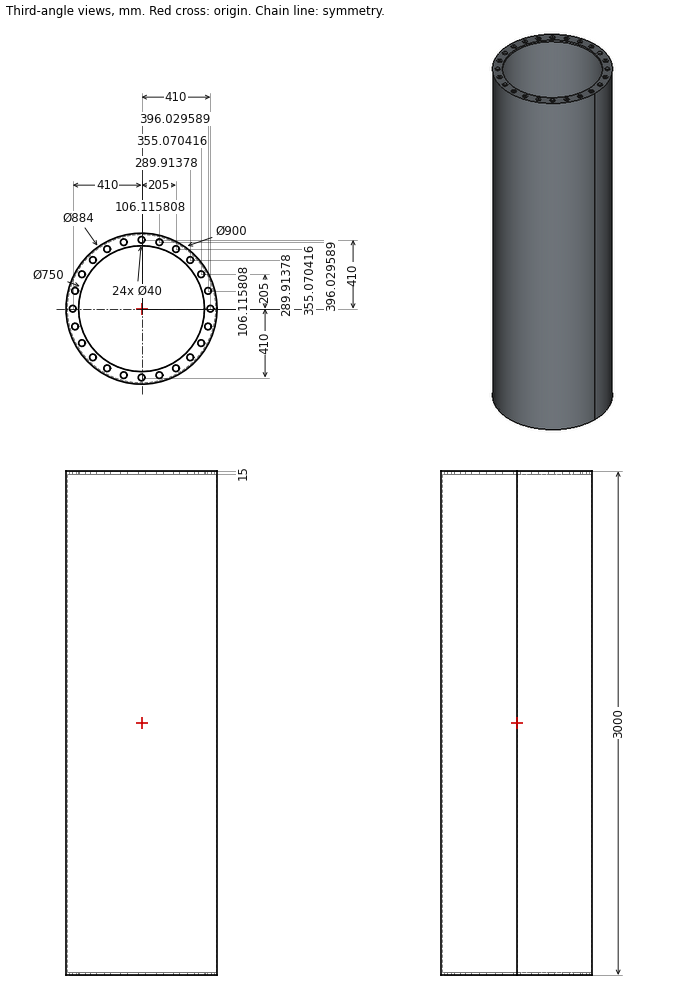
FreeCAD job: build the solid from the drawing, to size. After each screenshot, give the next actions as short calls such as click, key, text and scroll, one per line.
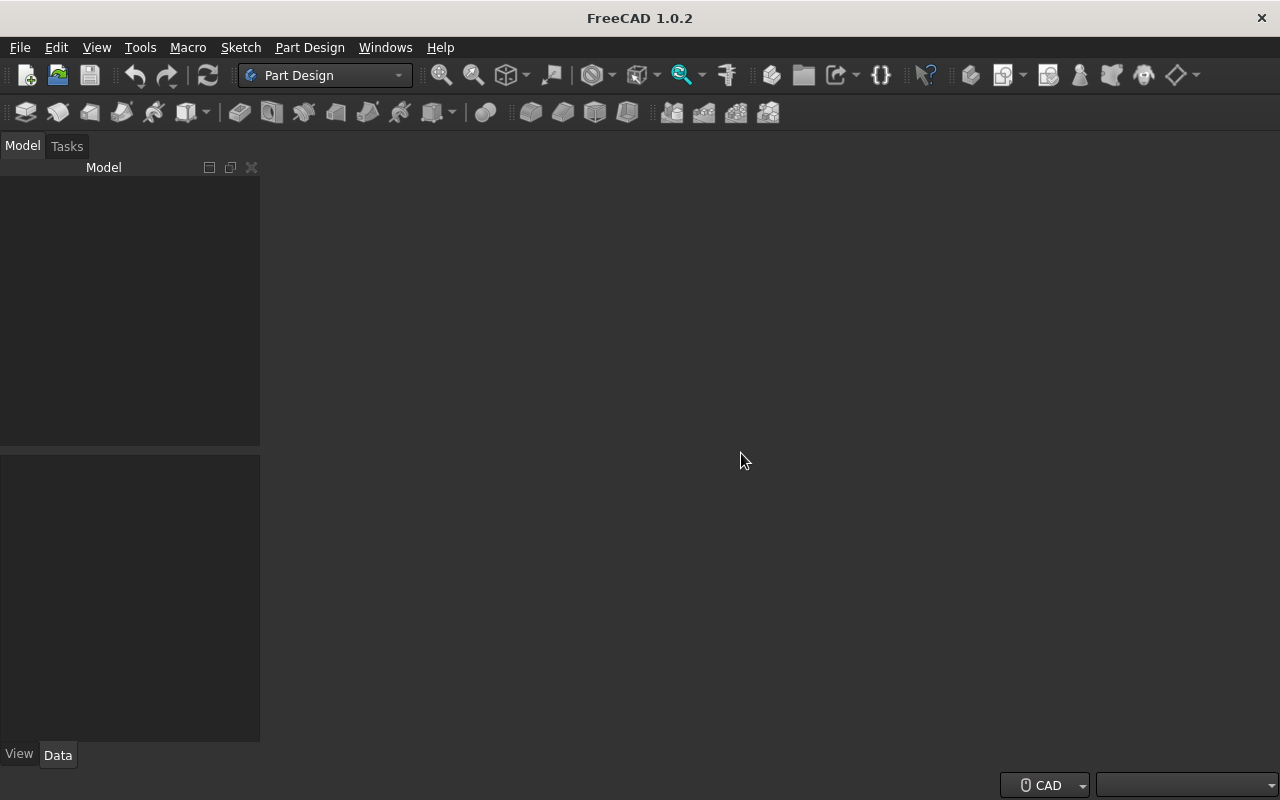
click(26, 76)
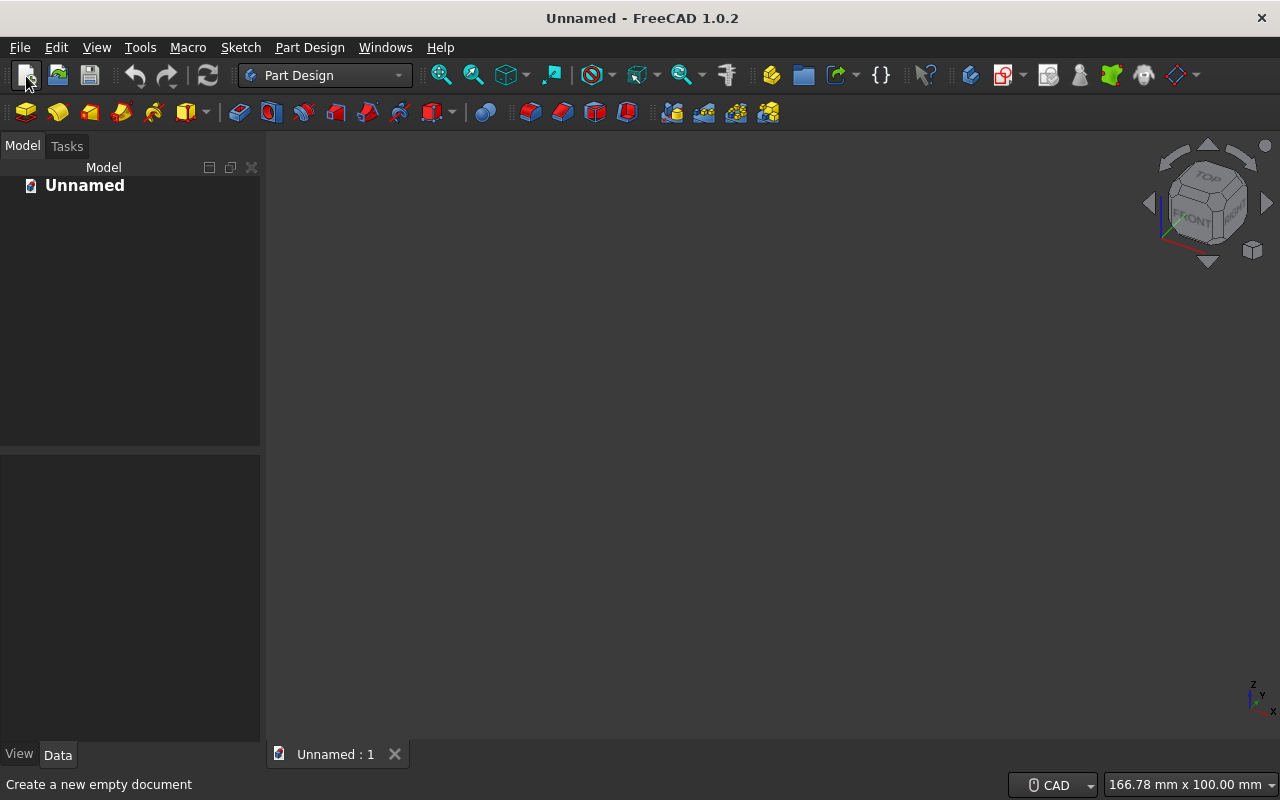
click(1004, 76)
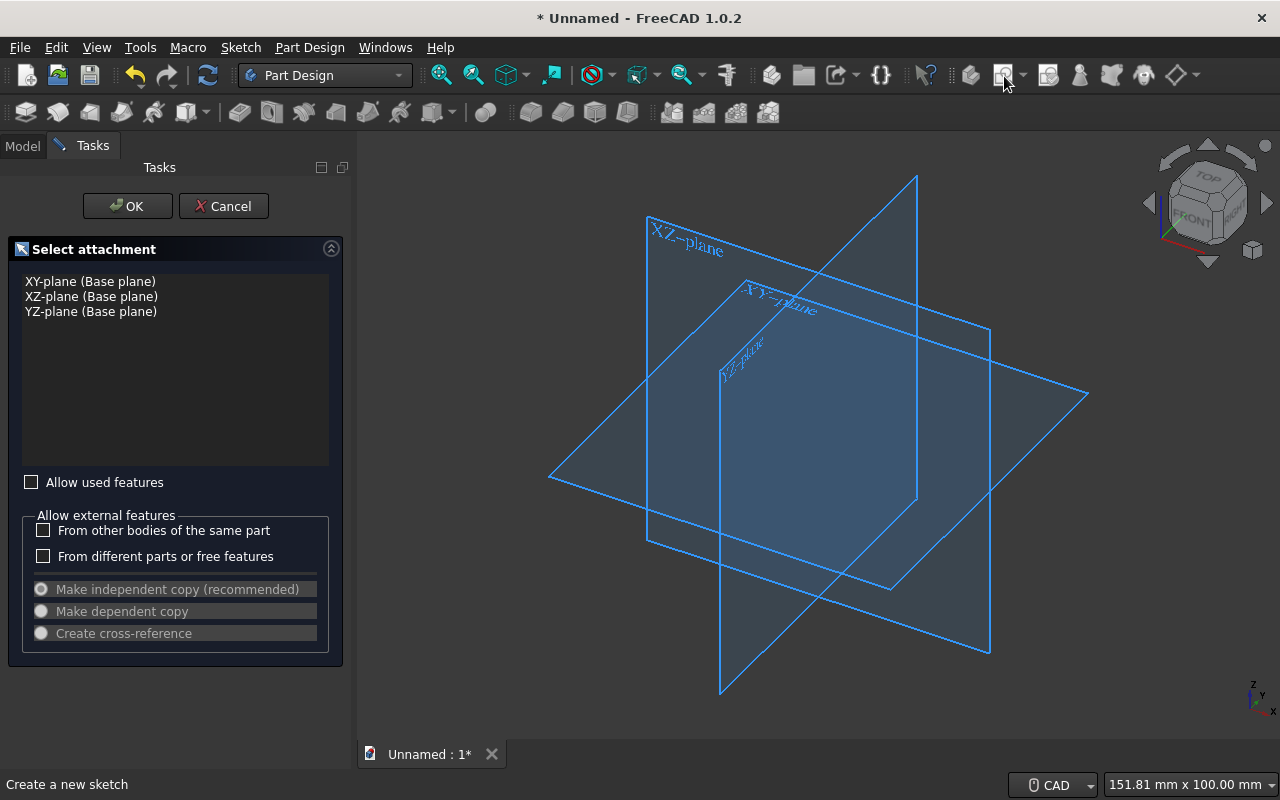
click(82, 282)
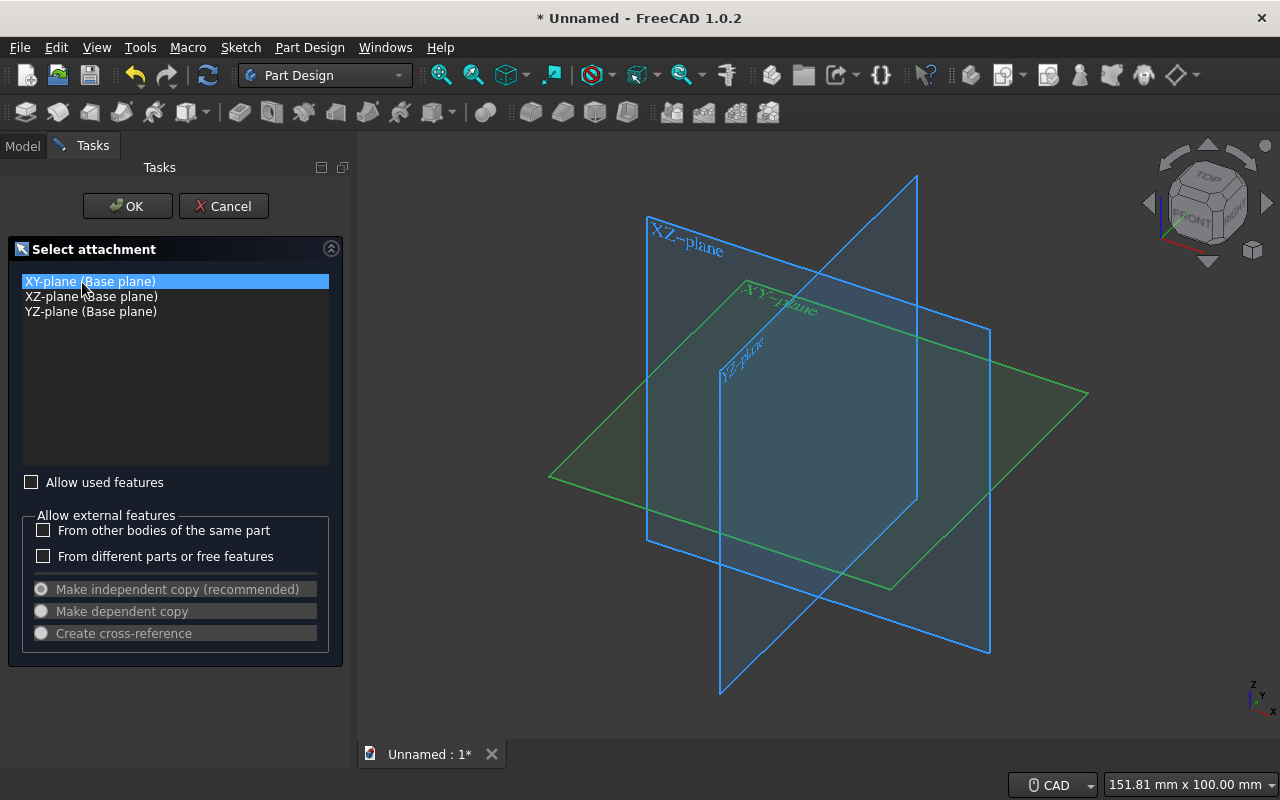
click(128, 206)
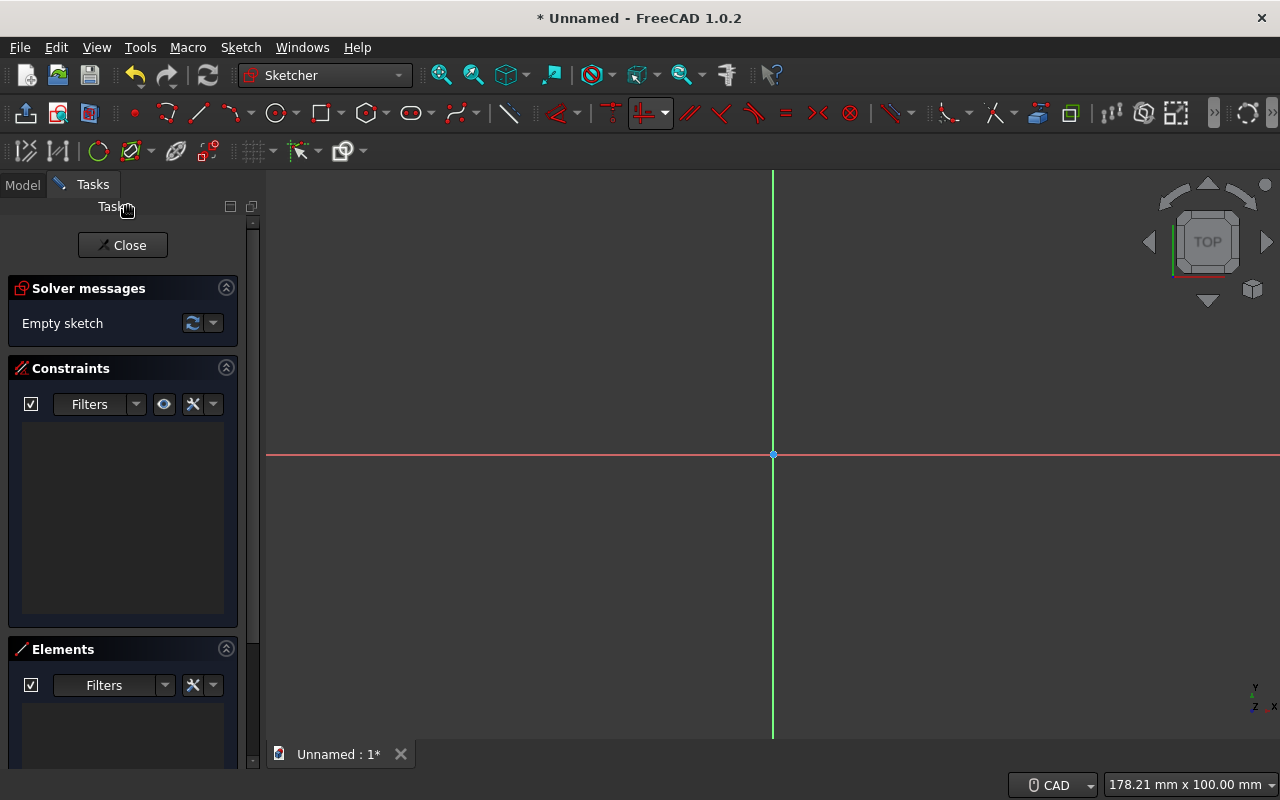
scroll(699, 454, down, 13)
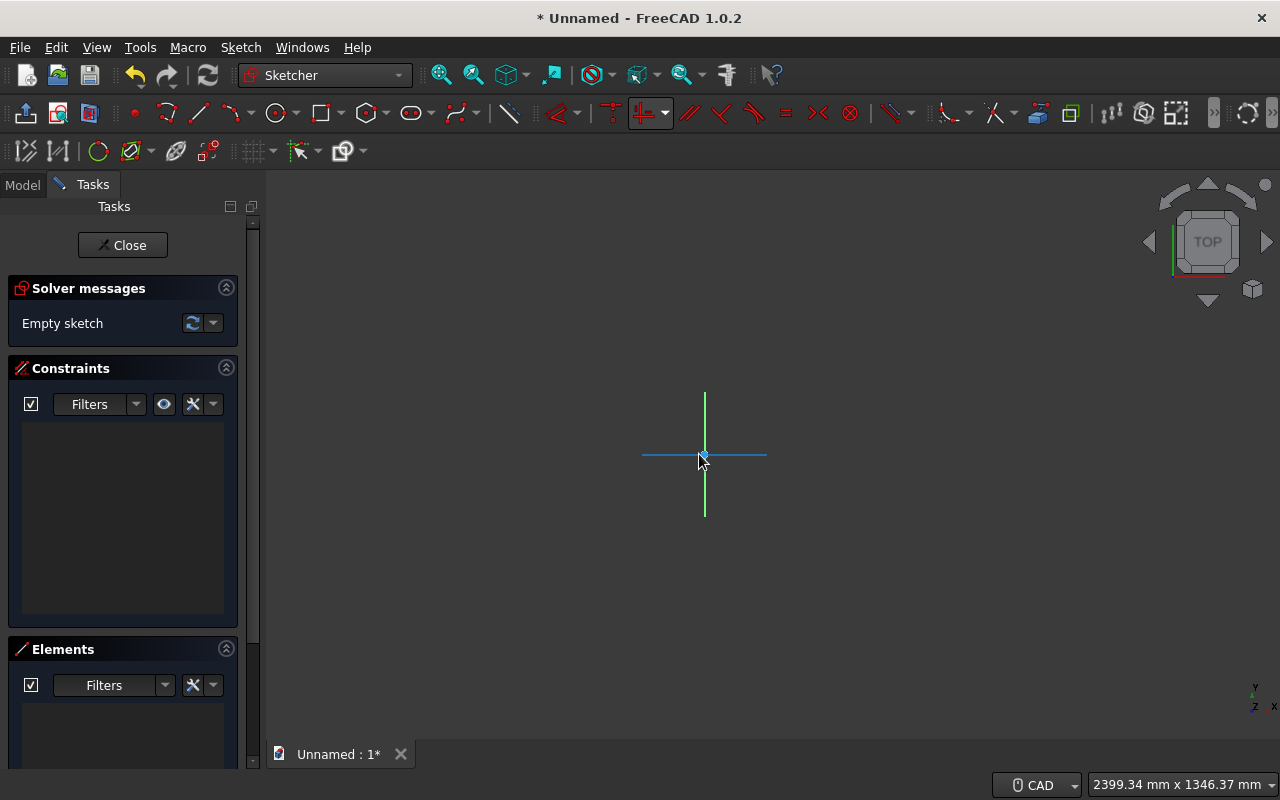
click(276, 114)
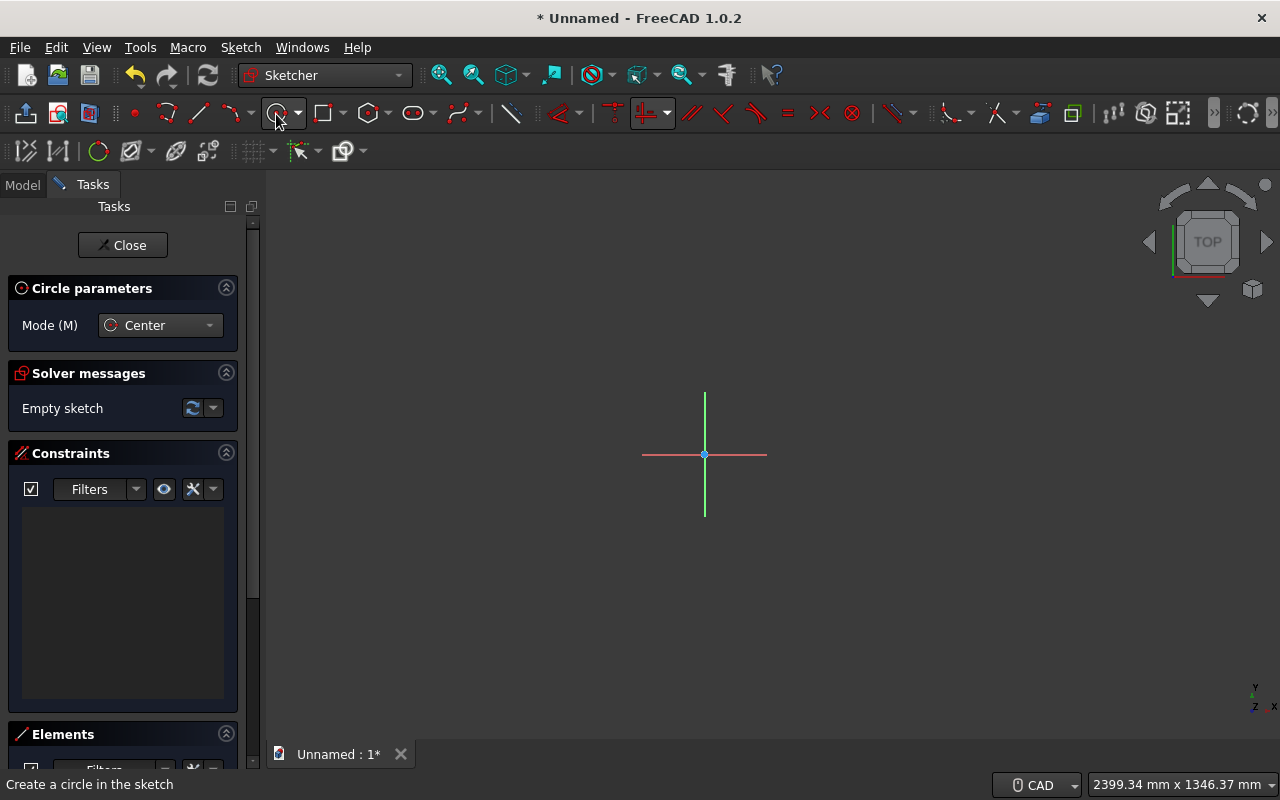
click(705, 454)
move(839, 320)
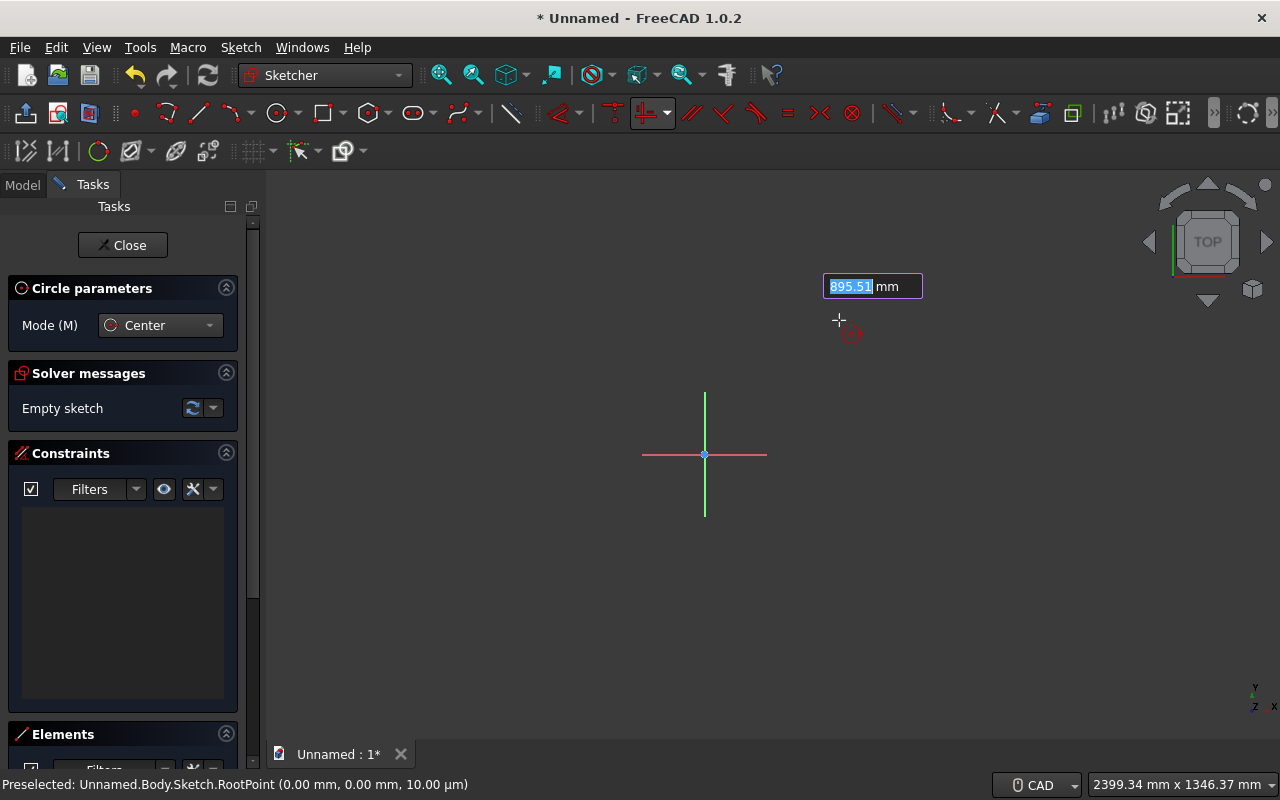
text(900)
key(Return)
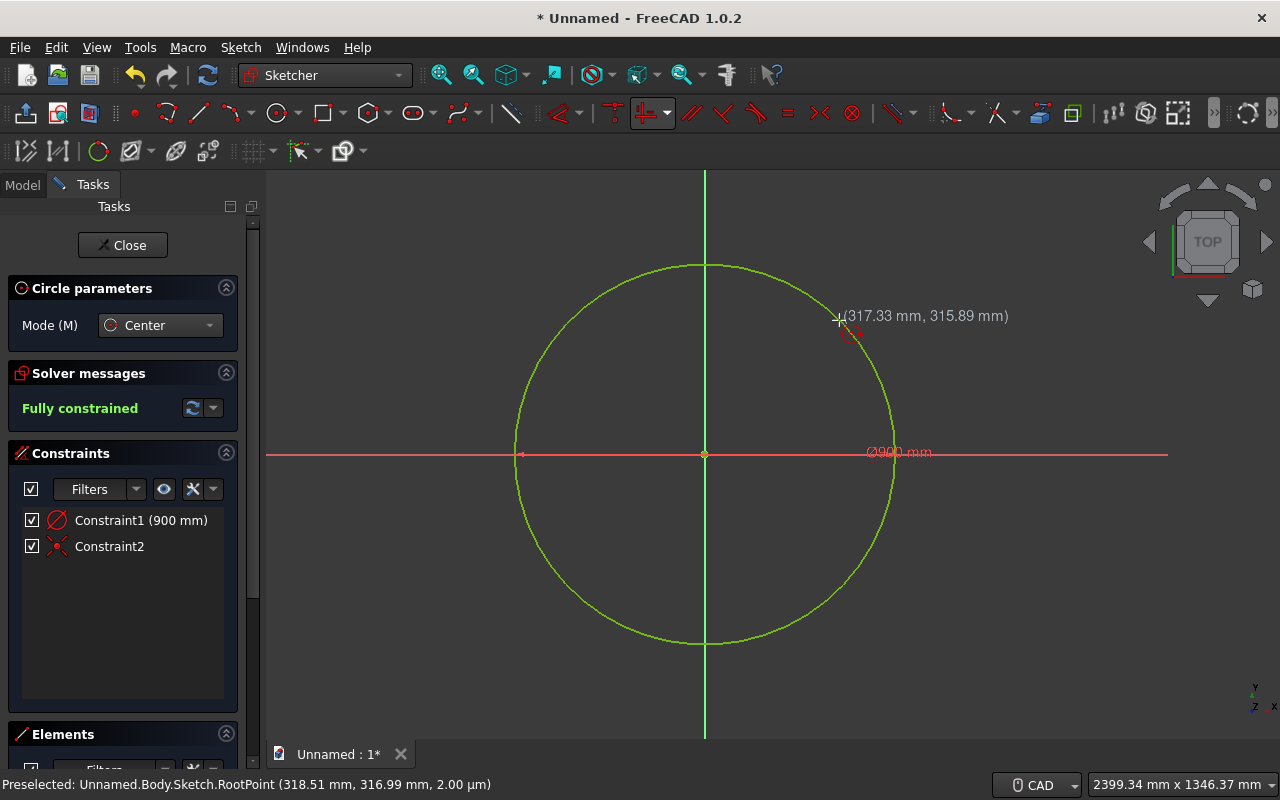
click(705, 454)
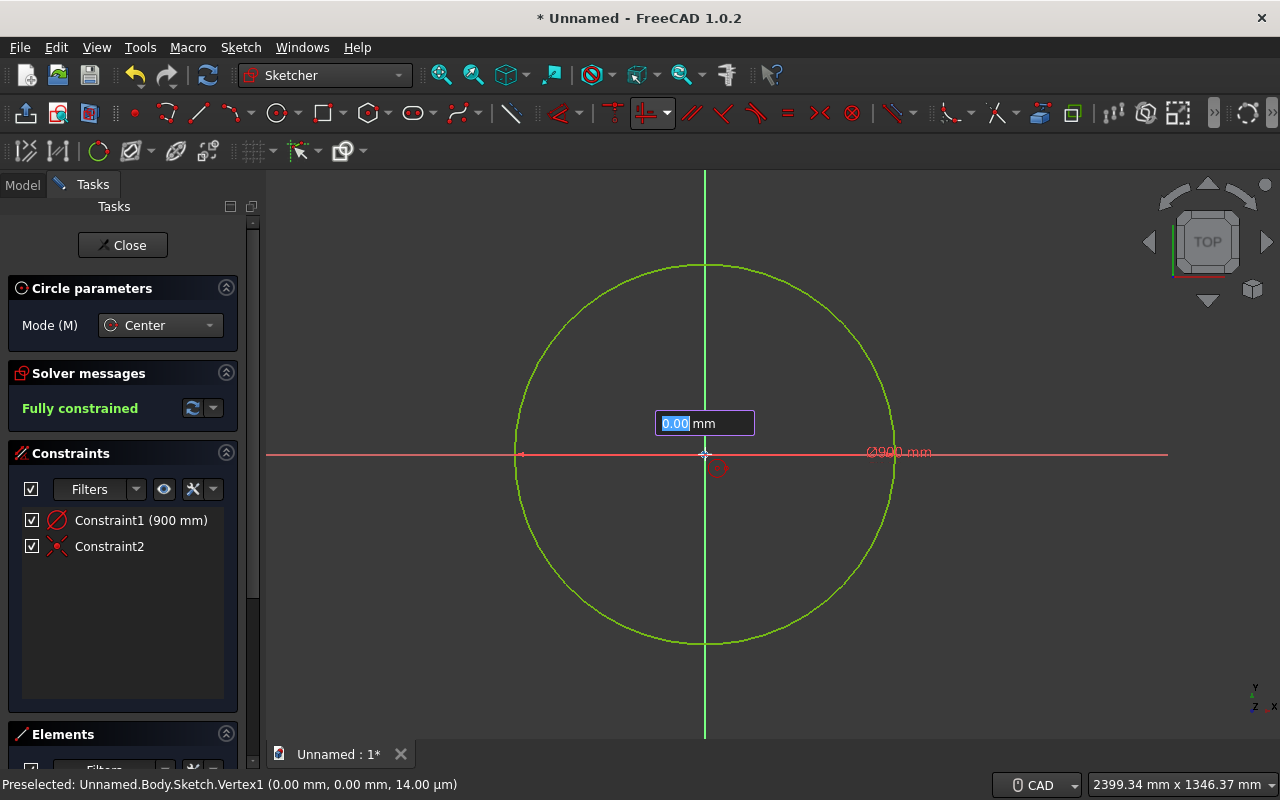
scroll(769, 279, up, 8)
move(766, 278)